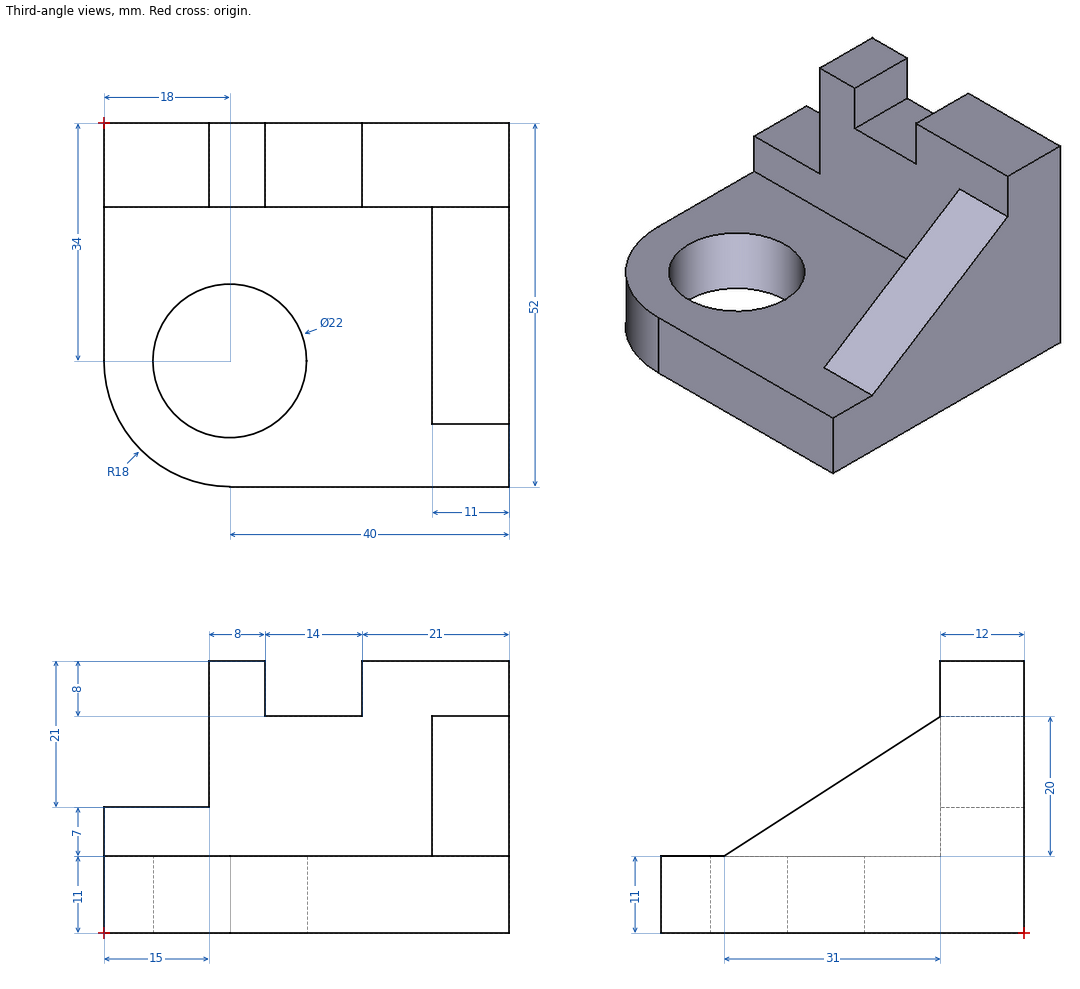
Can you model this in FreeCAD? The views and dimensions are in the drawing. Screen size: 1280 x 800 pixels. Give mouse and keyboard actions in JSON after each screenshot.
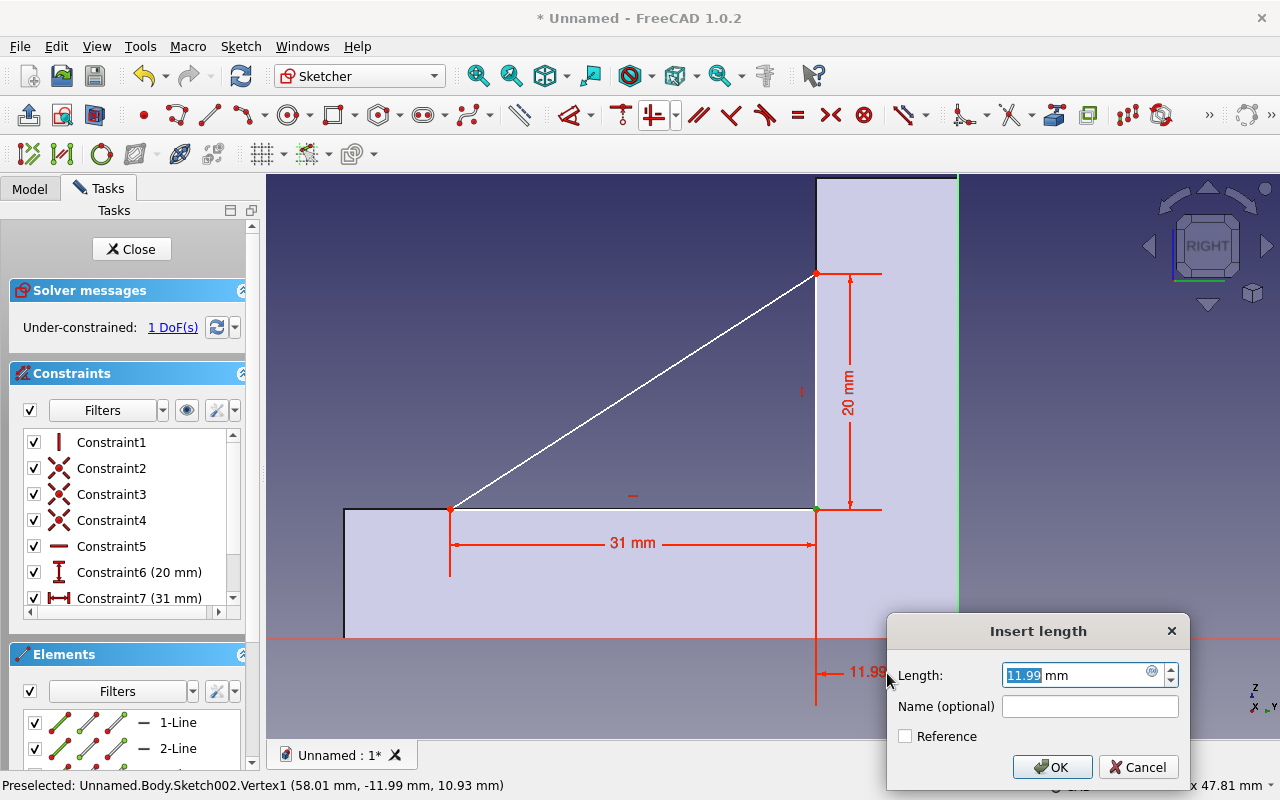
{"action": "type", "text": "12"}
{"action": "key", "text": "Return"}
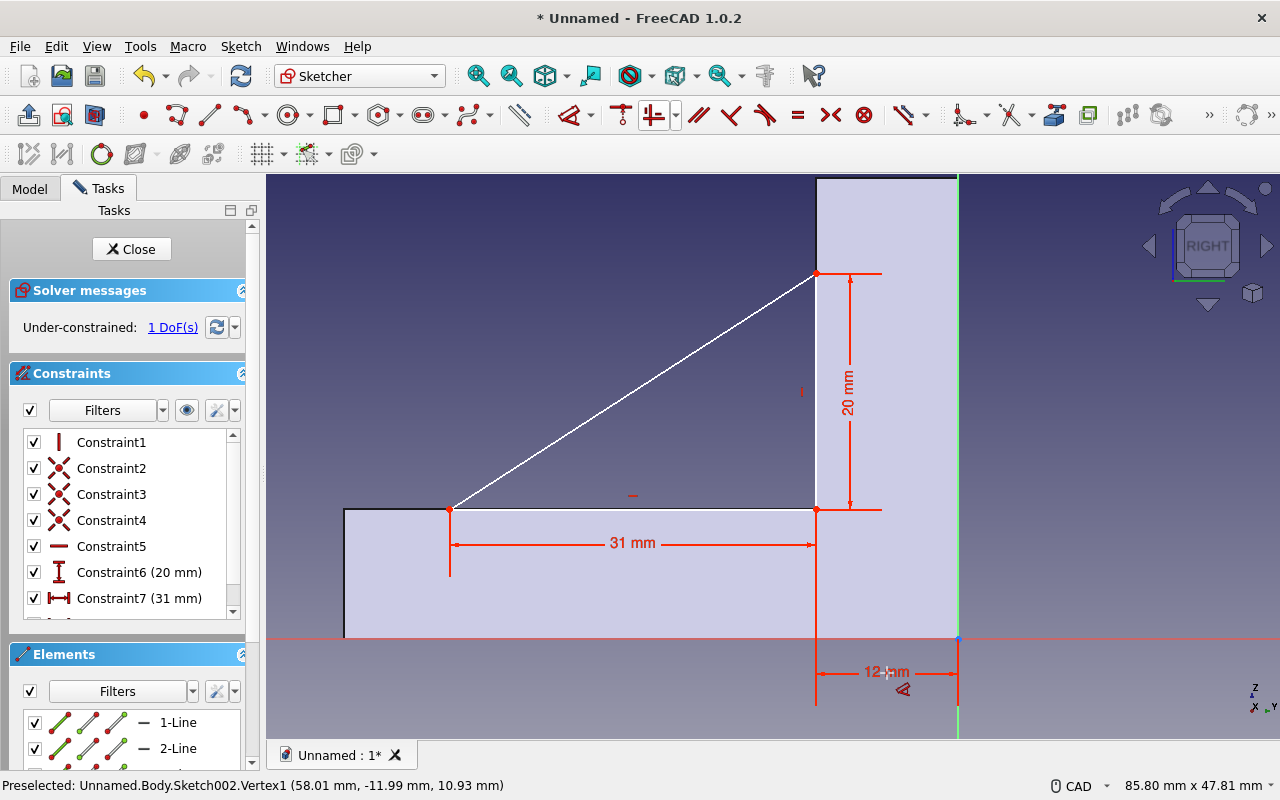
{"action": "left_click", "coordinate": [816, 510]}
{"action": "left_click", "coordinate": [992, 575]}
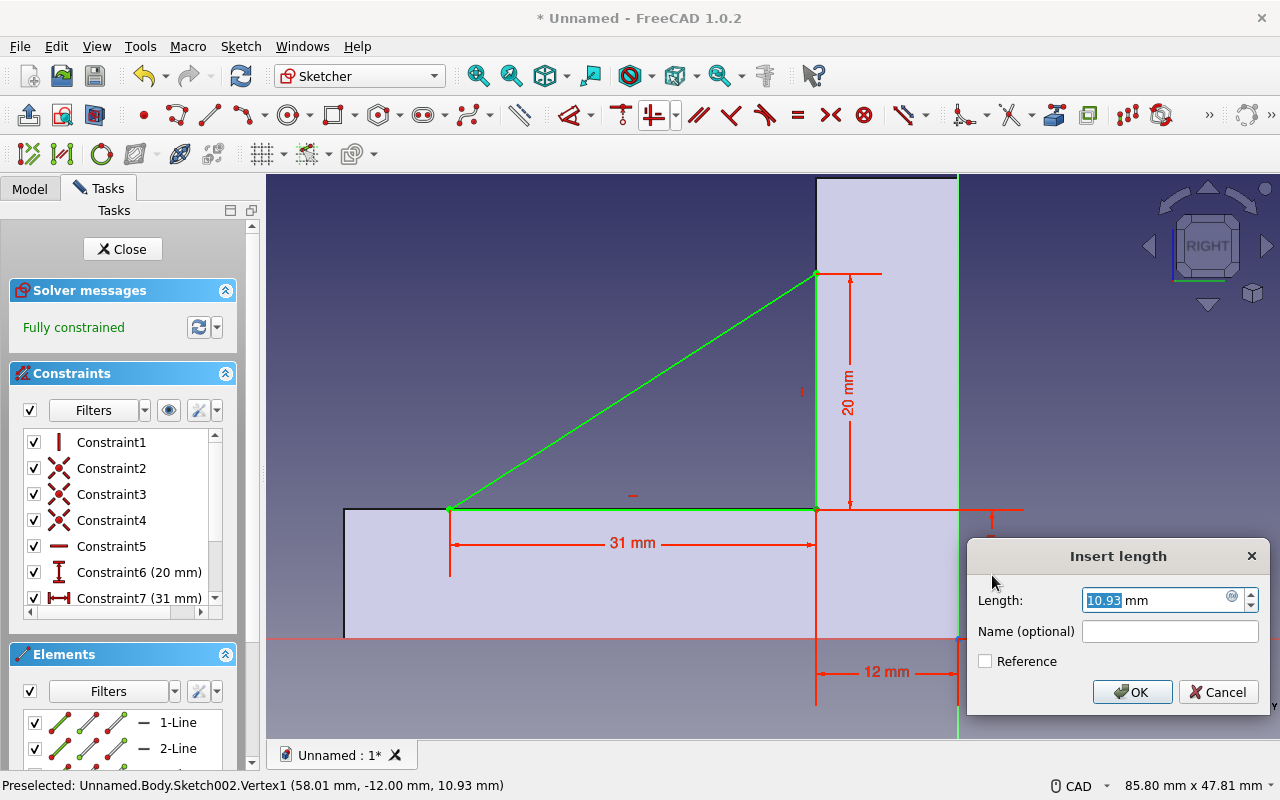
{"action": "type", "text": "11"}
{"action": "key", "text": "Return"}
{"action": "key", "text": "Escape"}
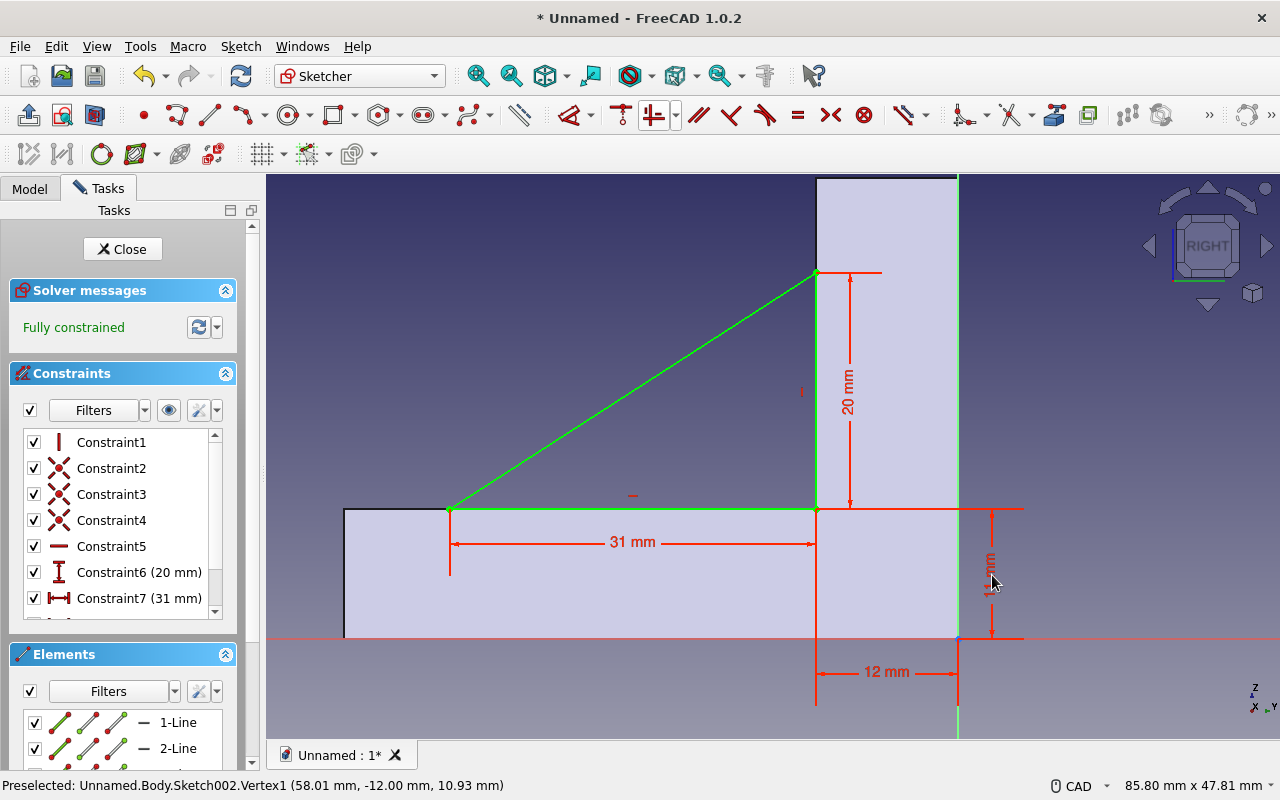
{"action": "left_click", "coordinate": [123, 249]}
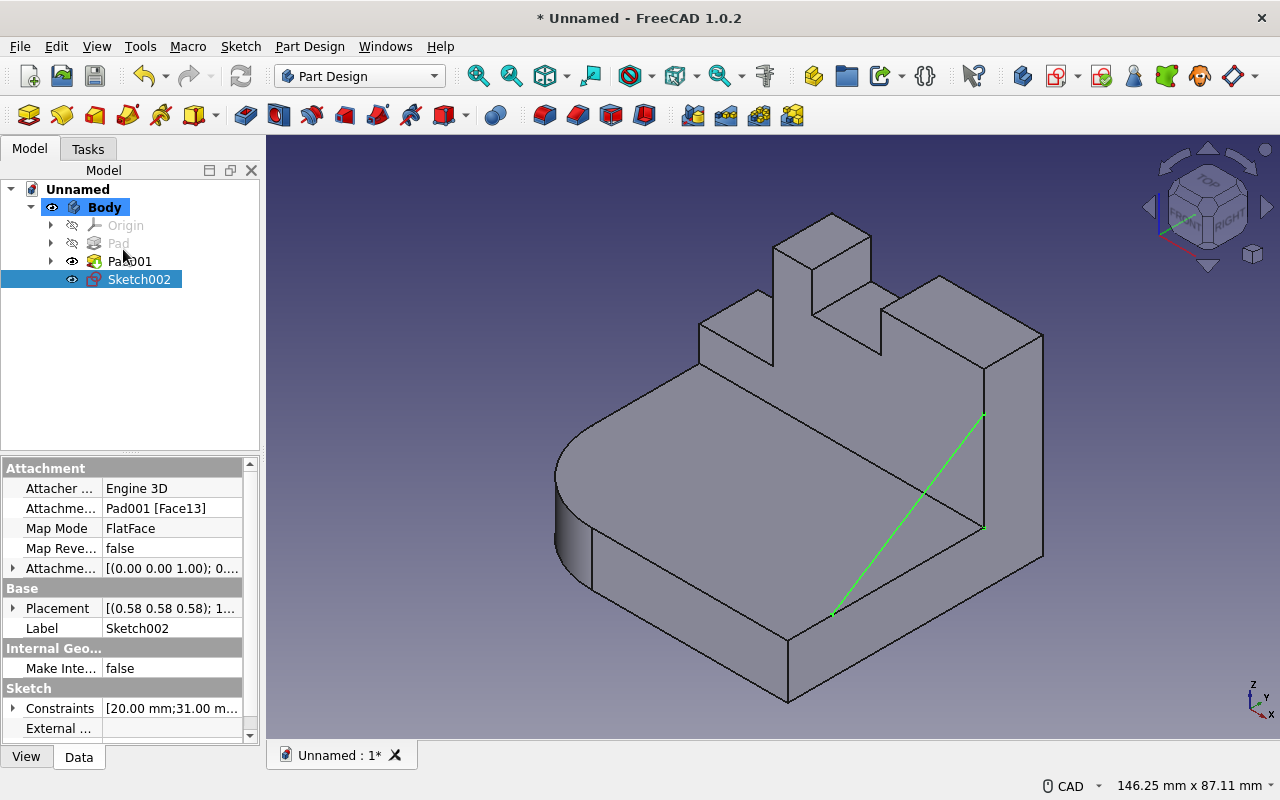
{"action": "left_click", "coordinate": [29, 116]}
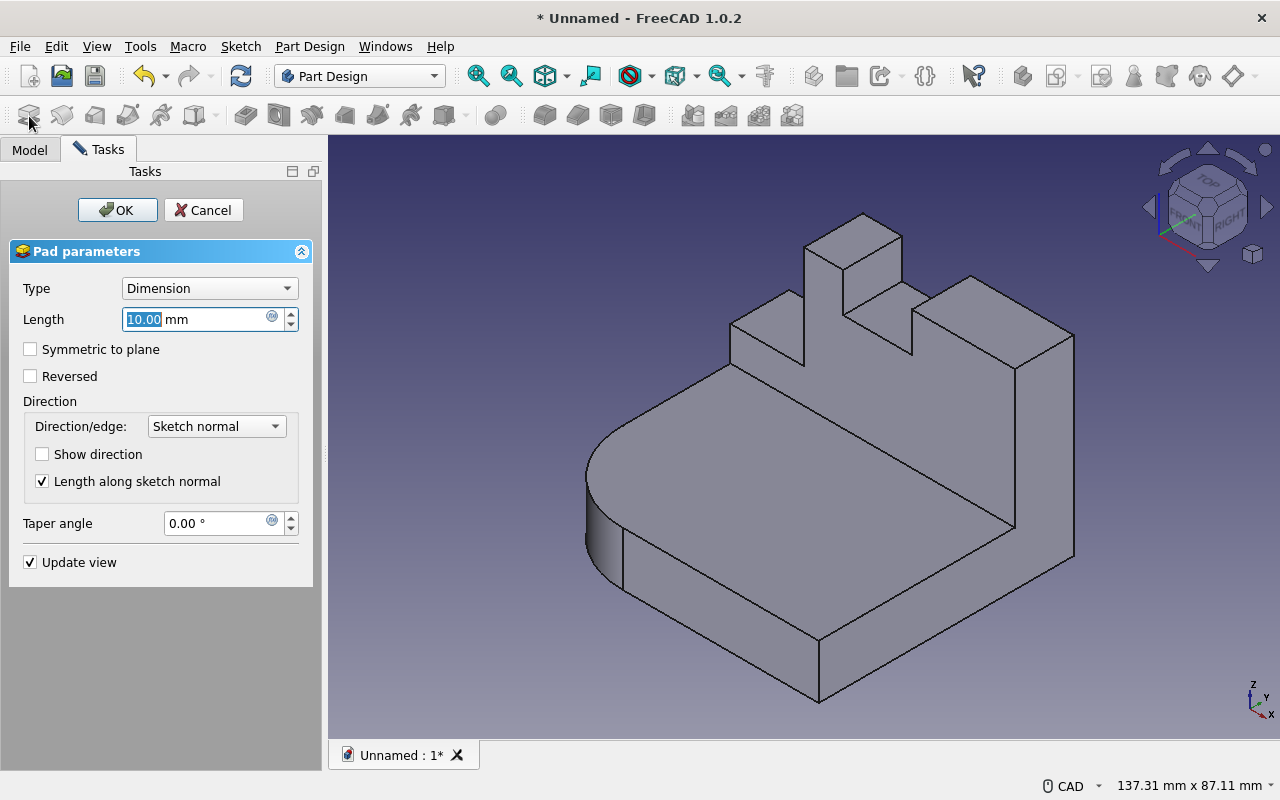
{"action": "type", "text": "11"}
{"action": "key", "text": "Tab"}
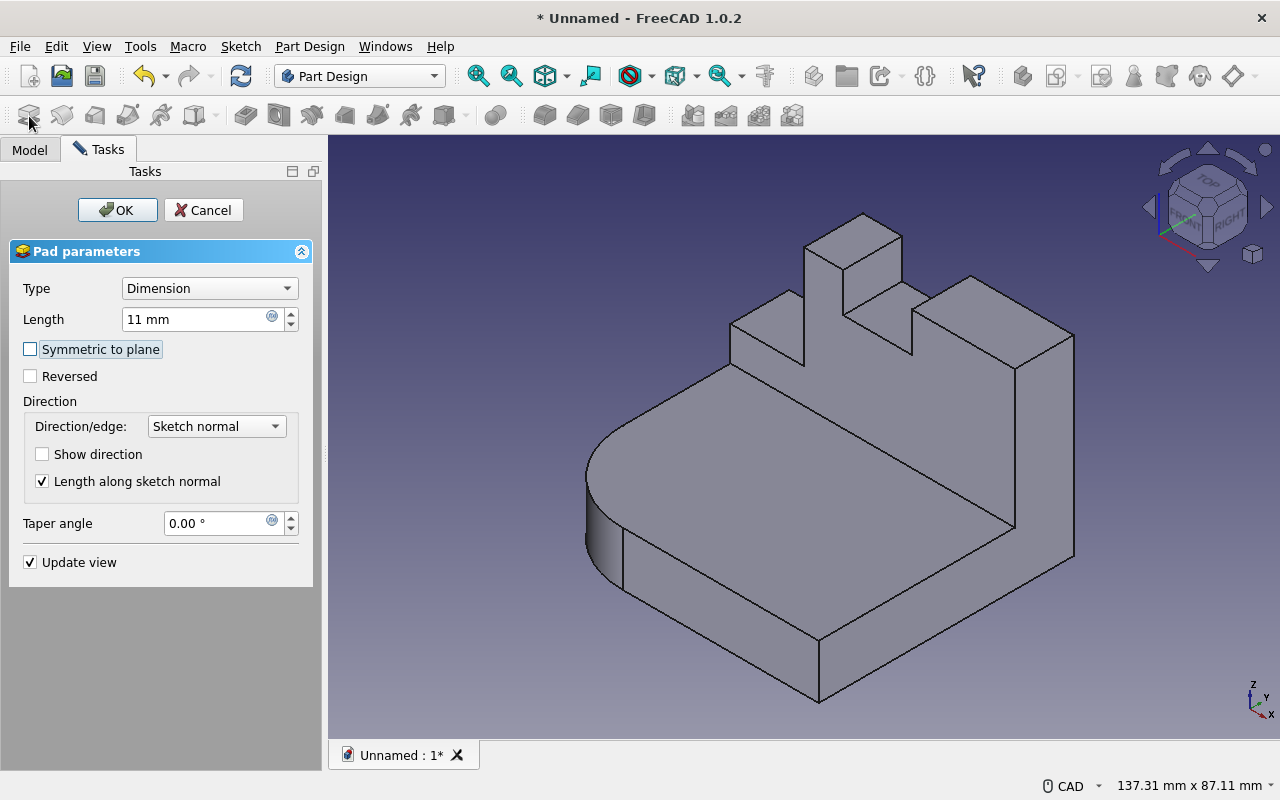
{"action": "left_click", "coordinate": [31, 376]}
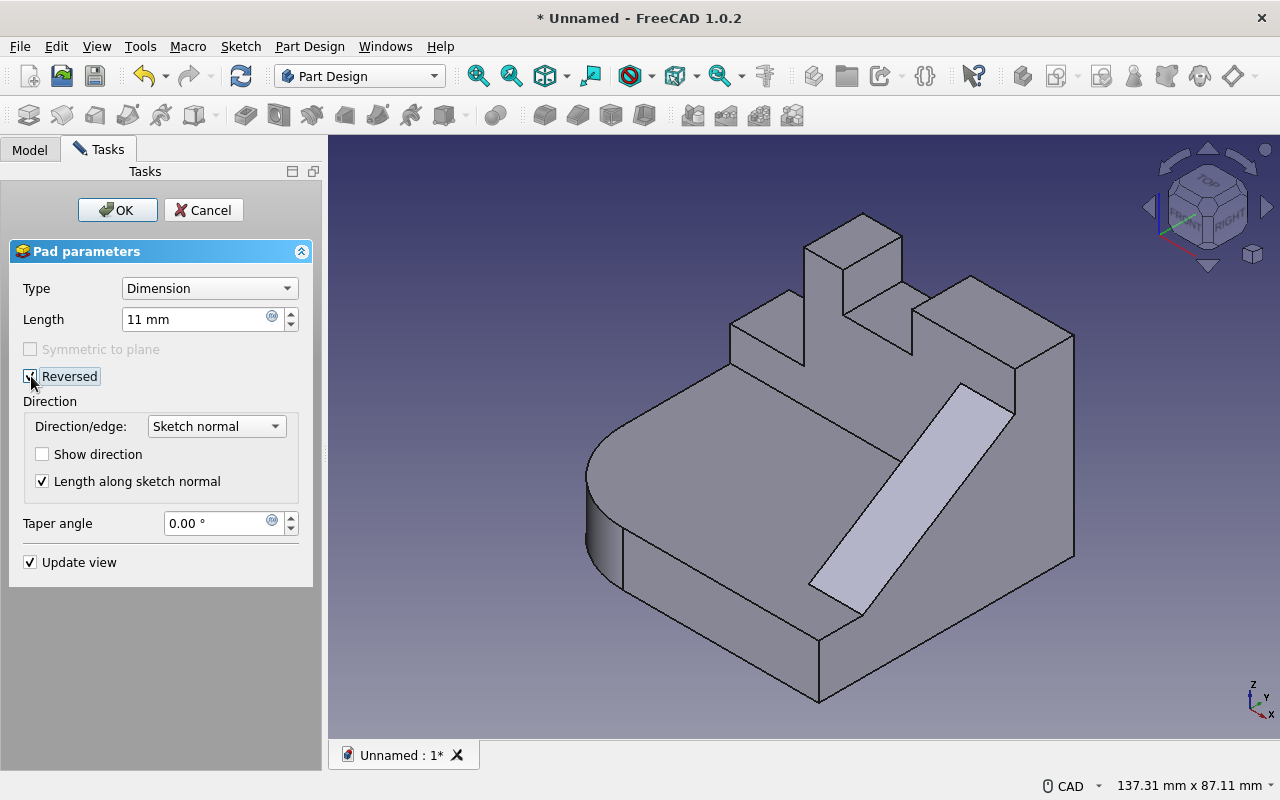
{"action": "left_click", "coordinate": [118, 210]}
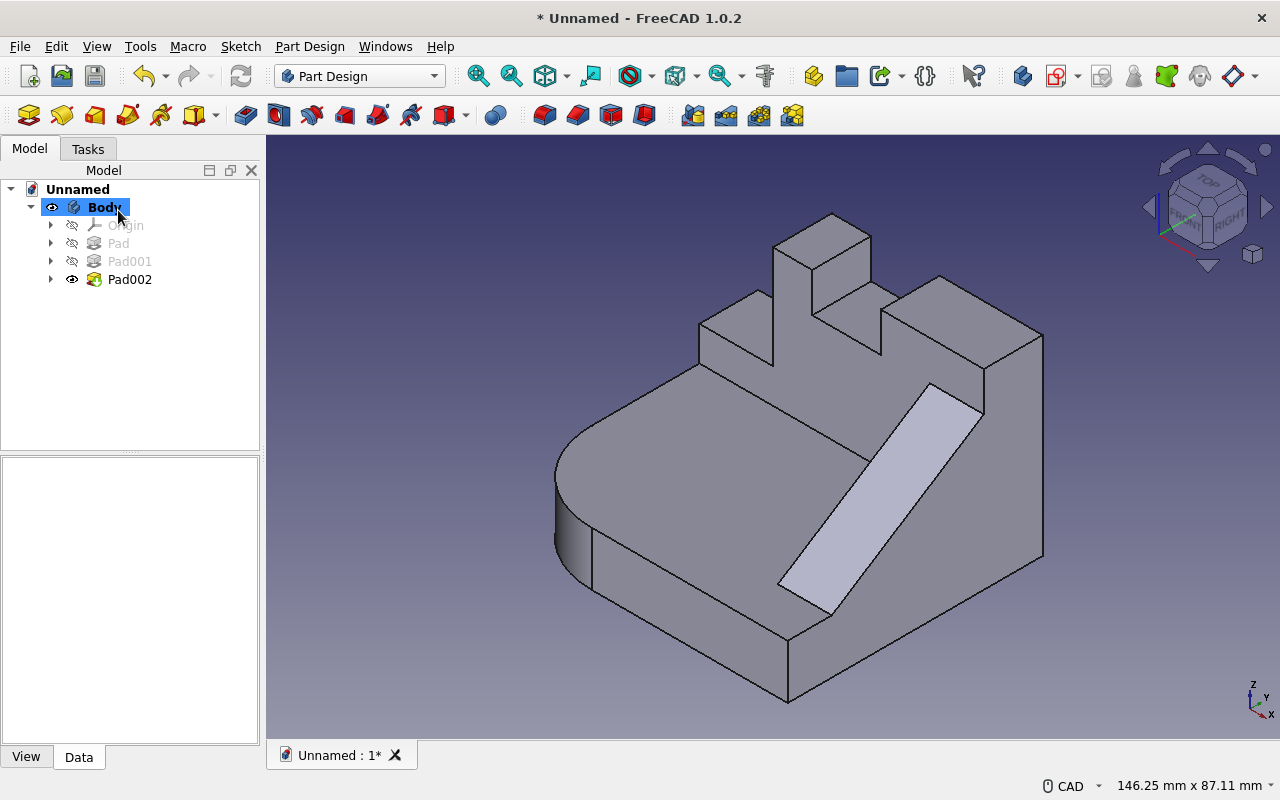
{"action": "left_click", "coordinate": [703, 478]}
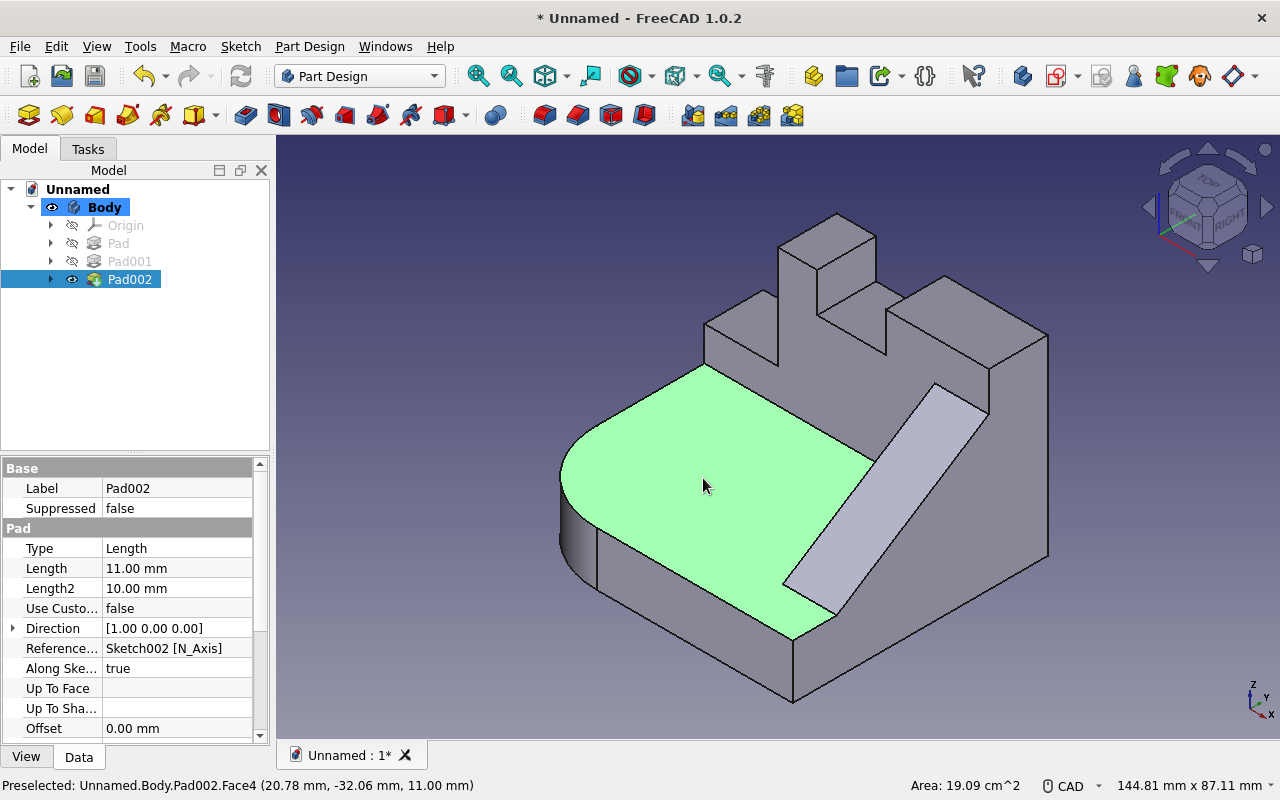
{"action": "left_click", "coordinate": [1056, 76]}